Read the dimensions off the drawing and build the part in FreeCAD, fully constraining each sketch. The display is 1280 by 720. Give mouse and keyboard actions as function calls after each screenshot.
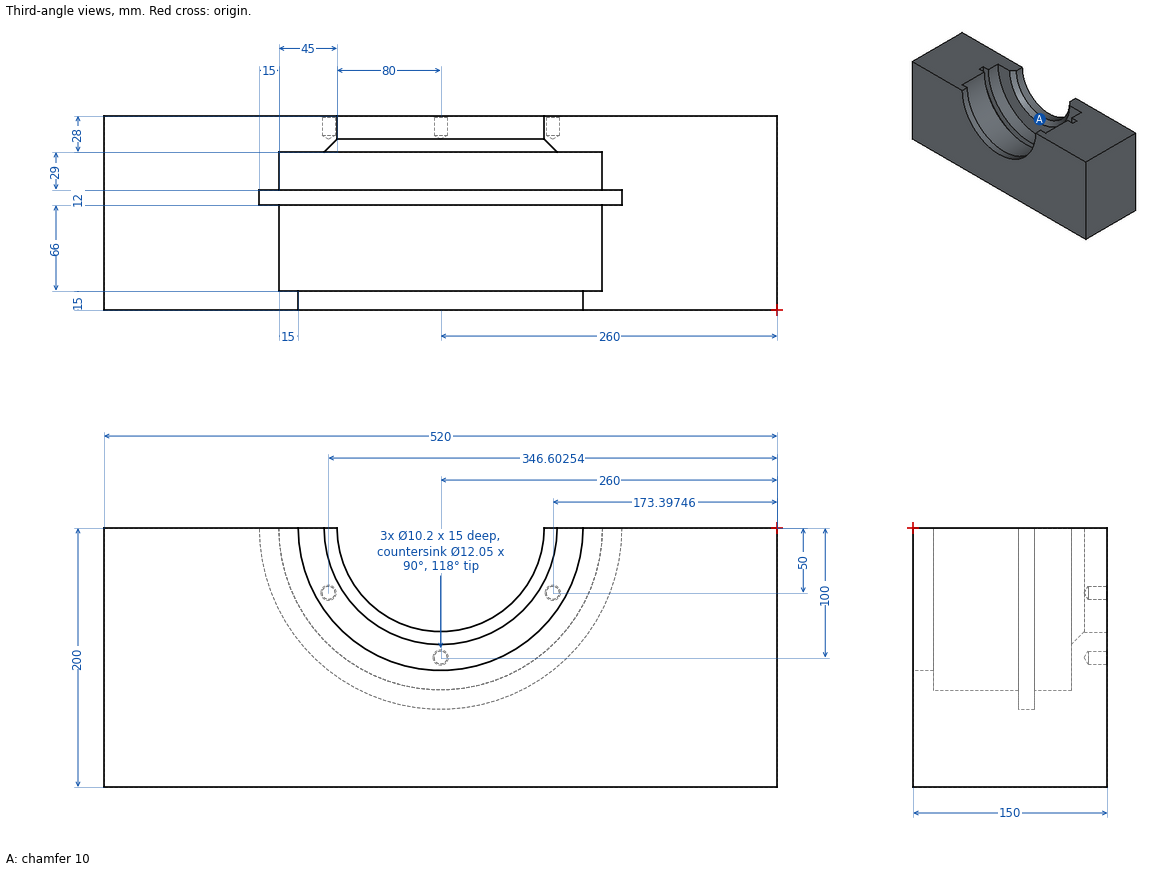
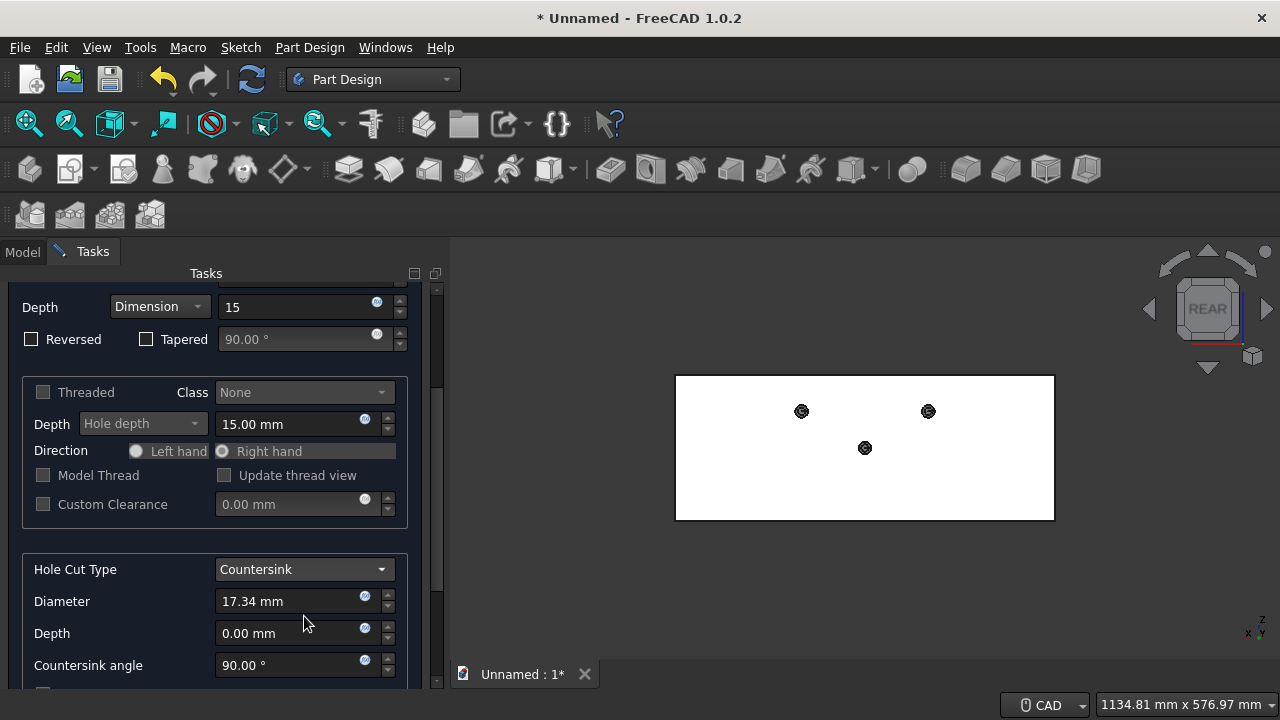
triple_click(298, 601)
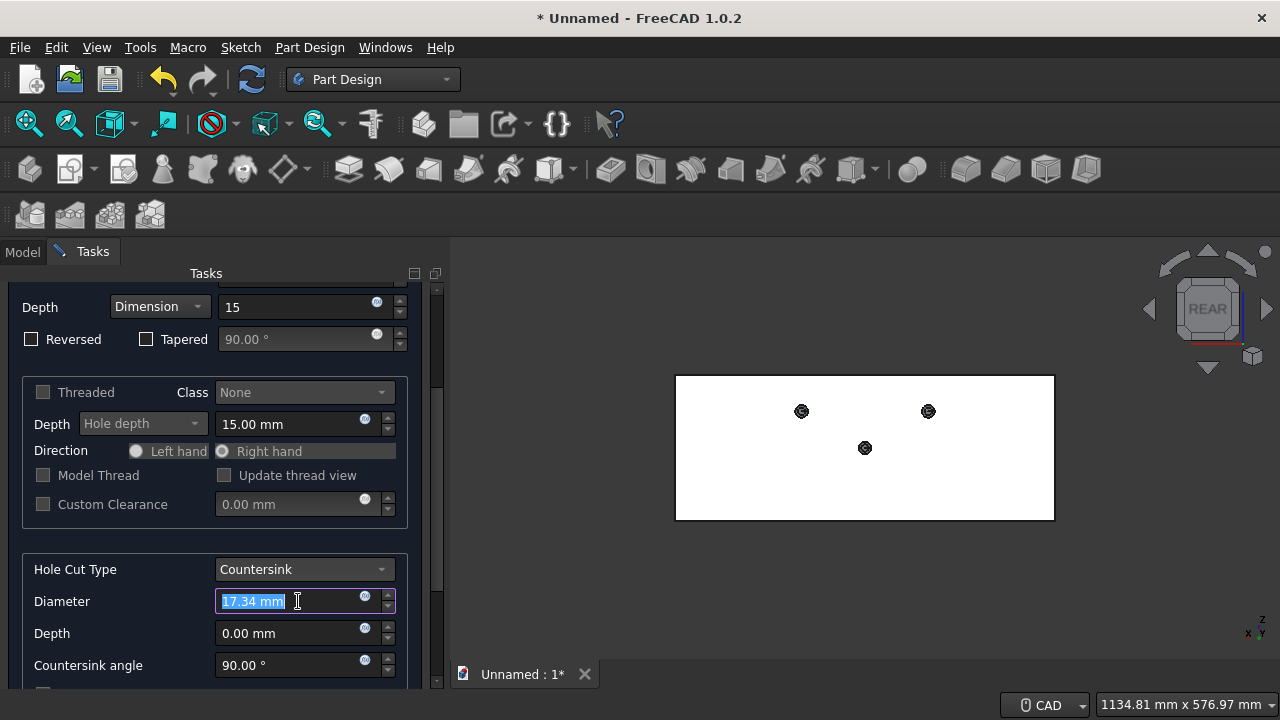
text(12.05)
key(Tab)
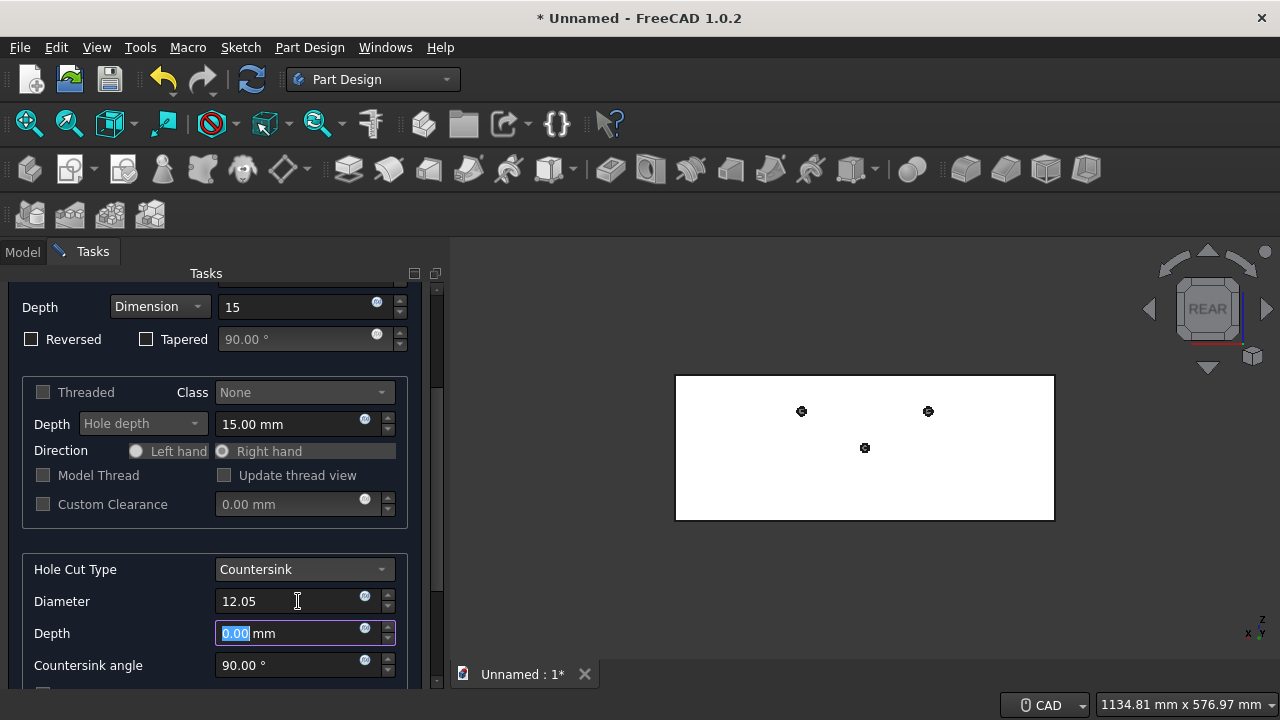
scroll(437, 486, up, 4)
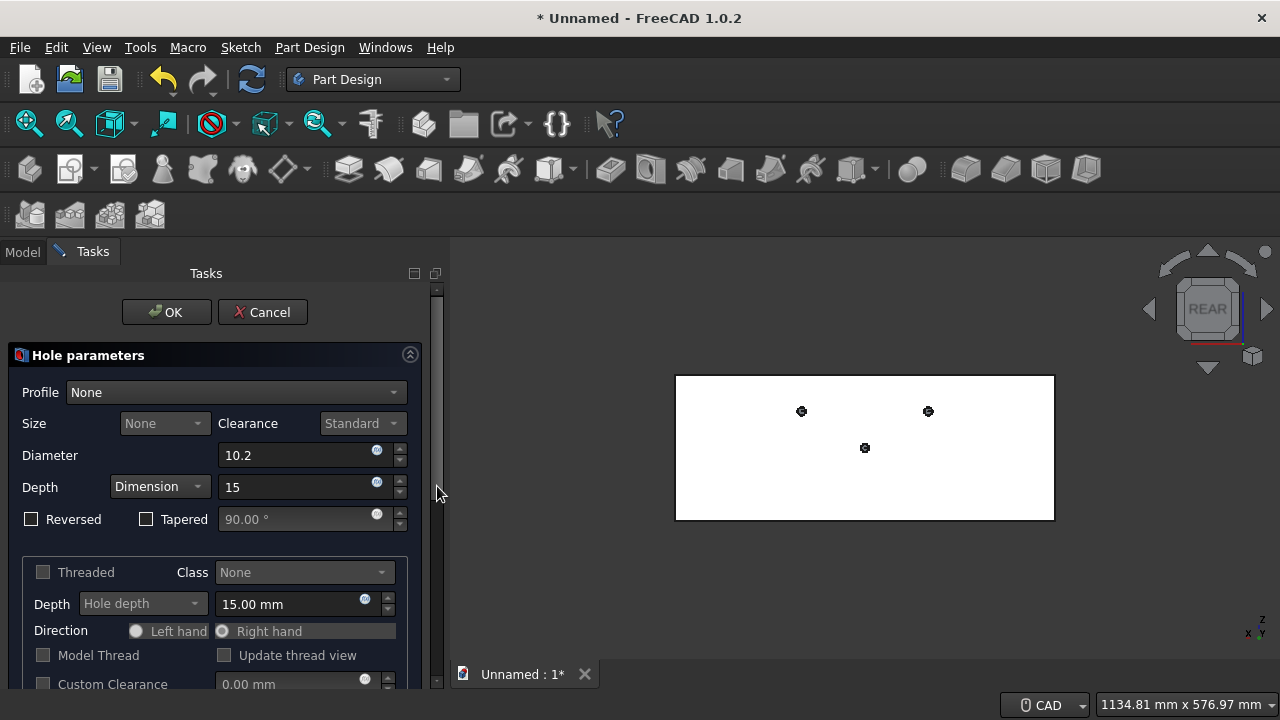
click(167, 312)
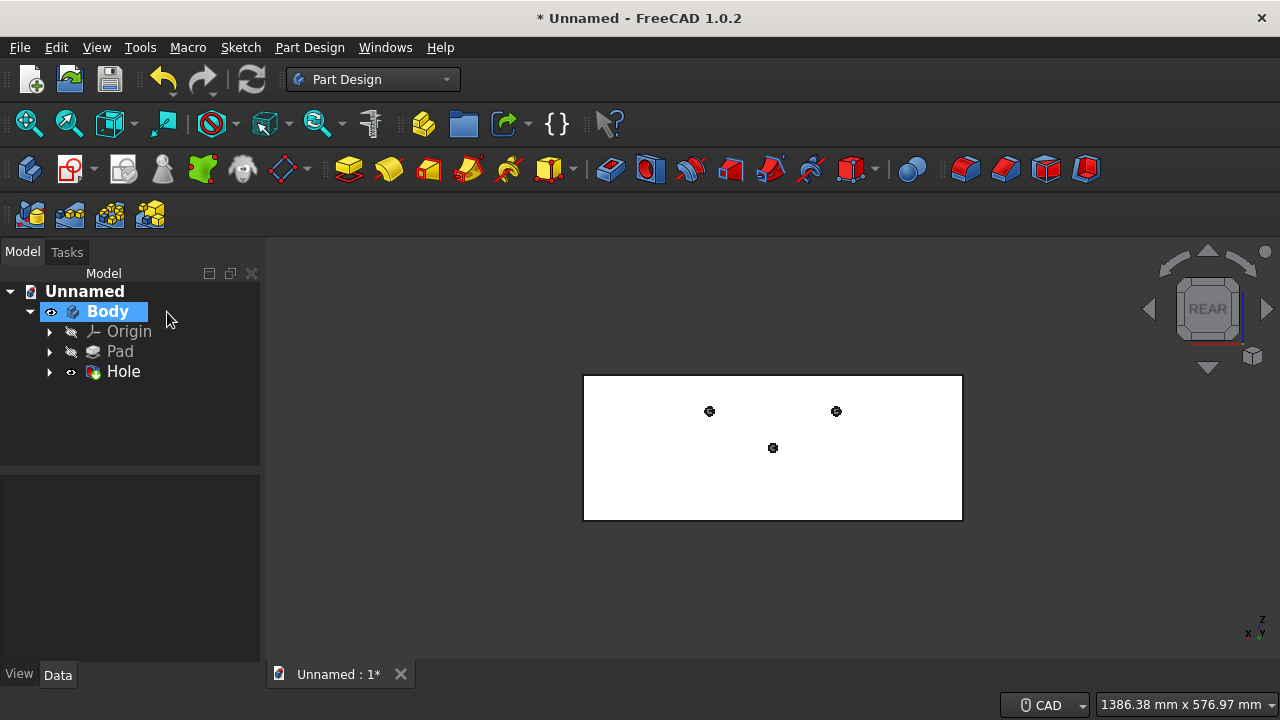
click(30, 124)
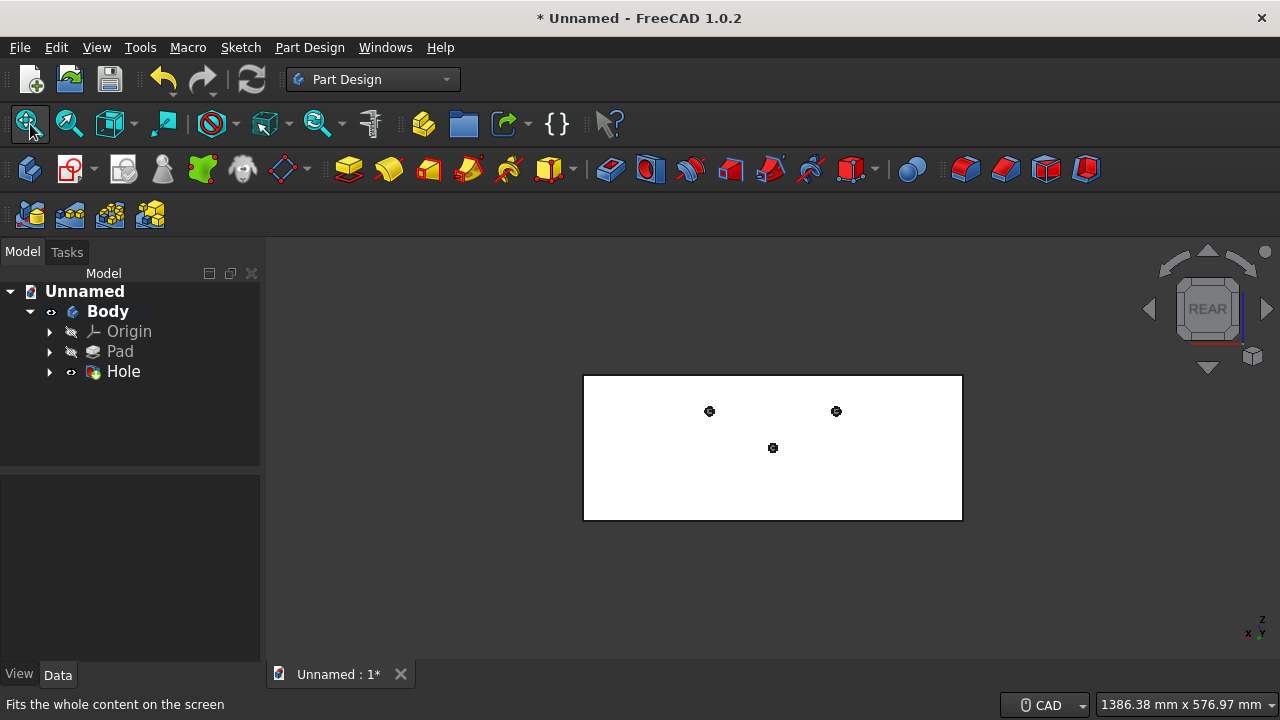
click(70, 170)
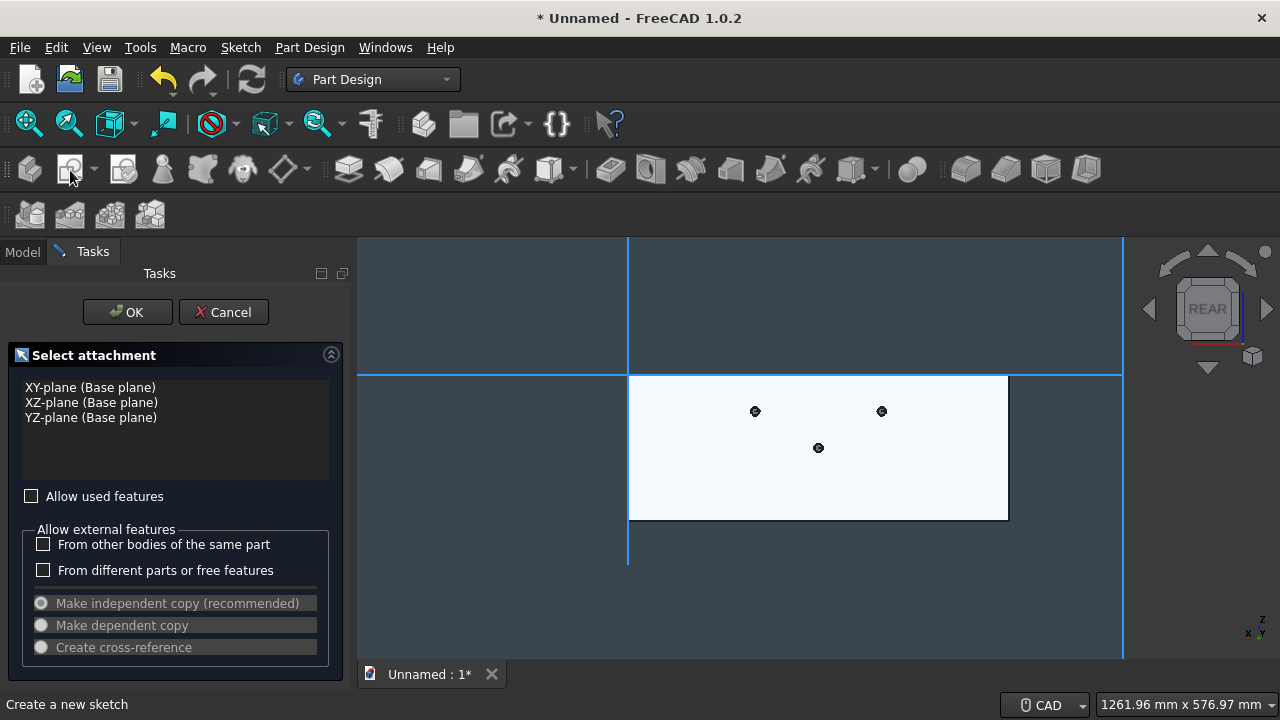
click(82, 388)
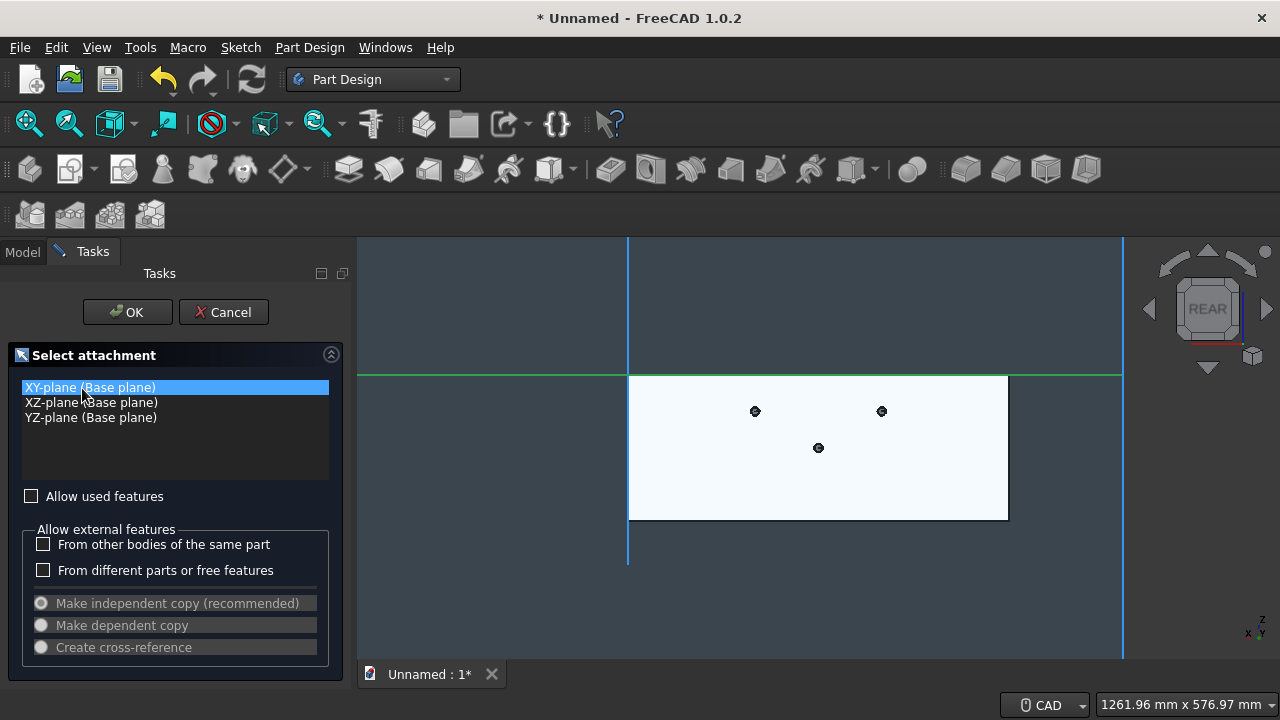
click(128, 312)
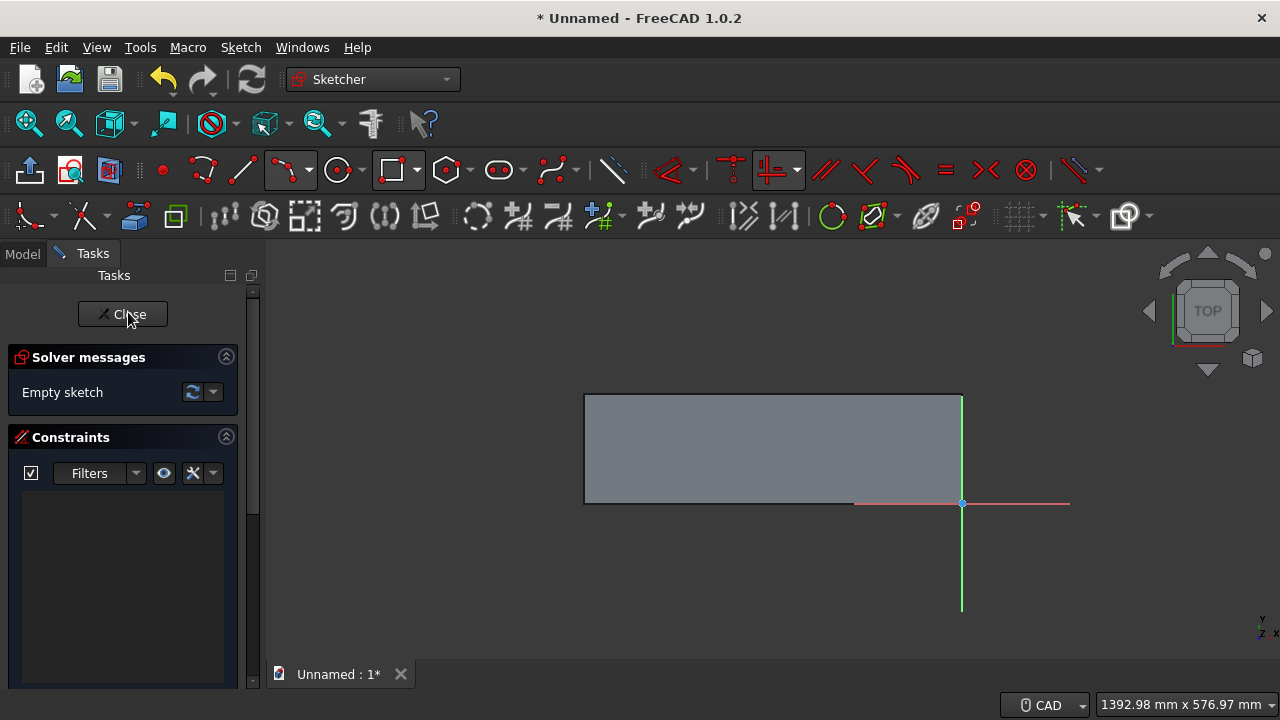
scroll(953, 401, up, 3)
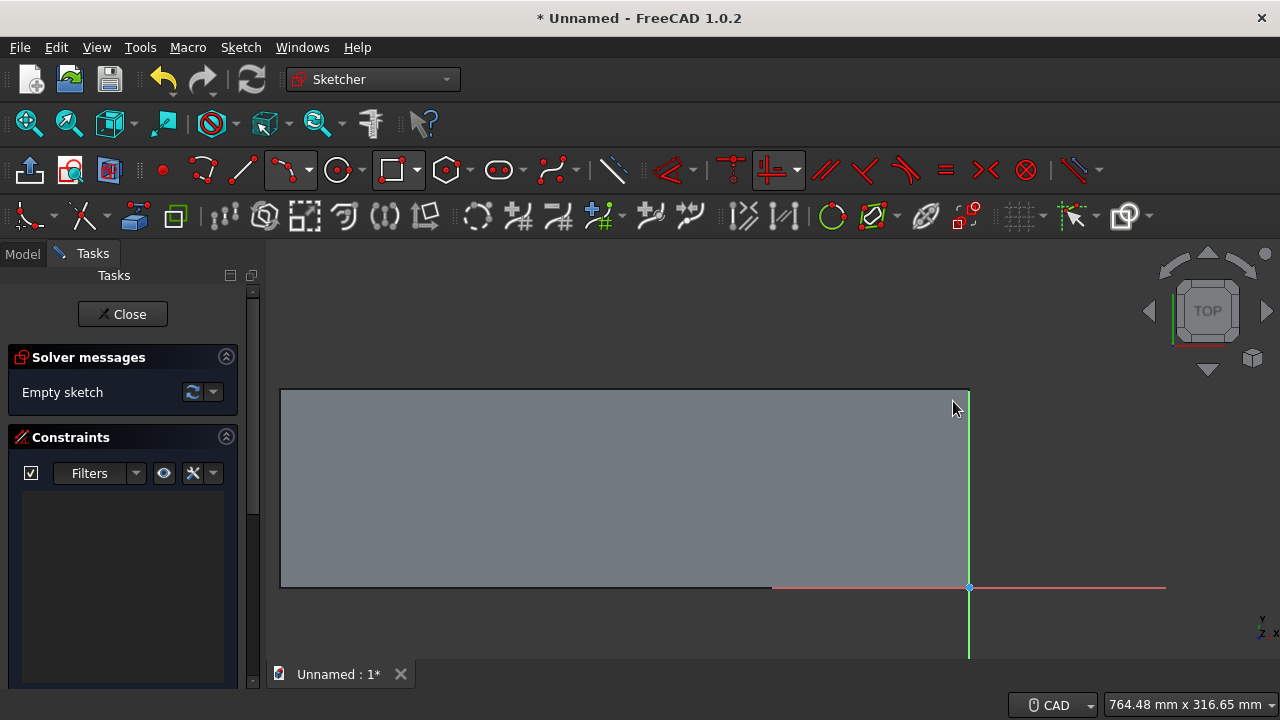
click(204, 170)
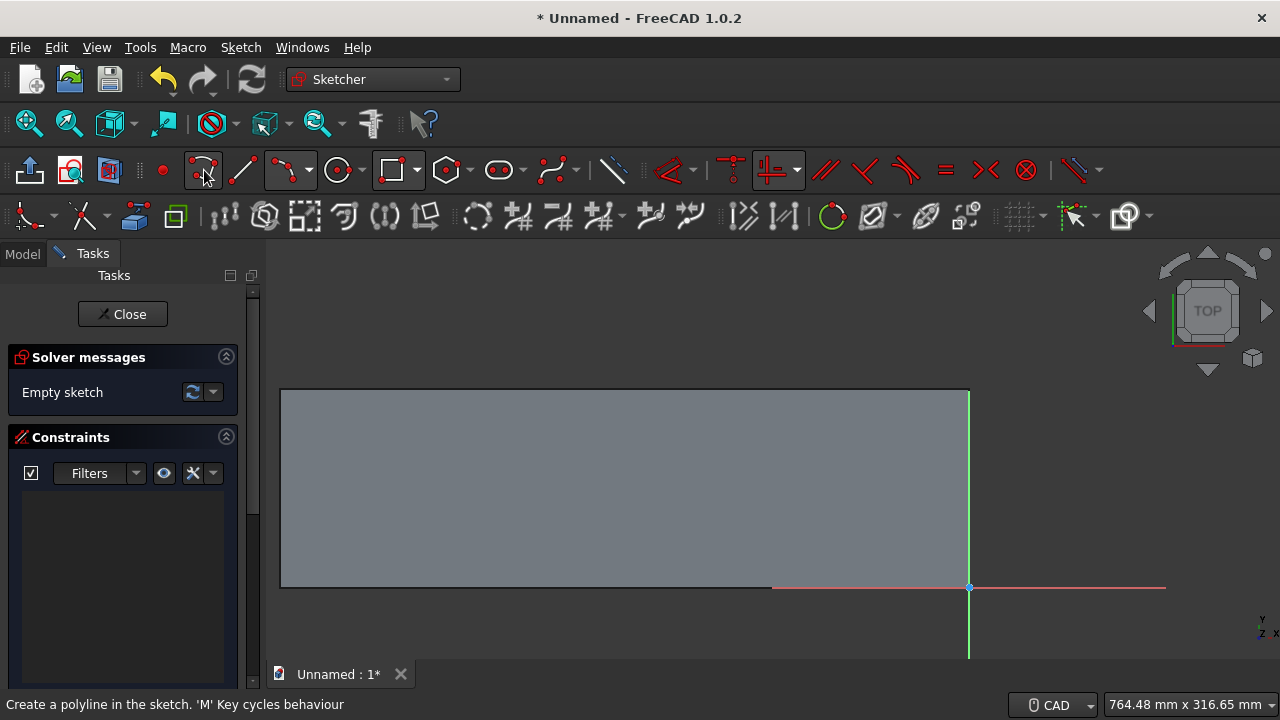
click(624, 588)
click(624, 389)
click(518, 389)
click(518, 426)
click(459, 426)
click(459, 464)
click(439, 464)
click(439, 480)
click(459, 480)
click(459, 568)
click(479, 568)
click(479, 579)
click(624, 589)